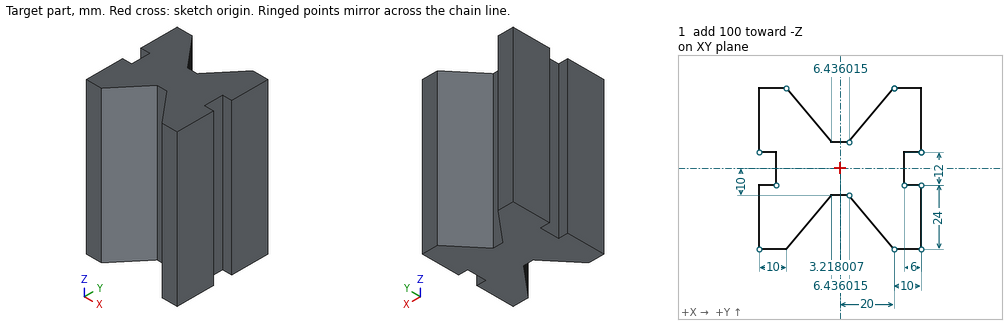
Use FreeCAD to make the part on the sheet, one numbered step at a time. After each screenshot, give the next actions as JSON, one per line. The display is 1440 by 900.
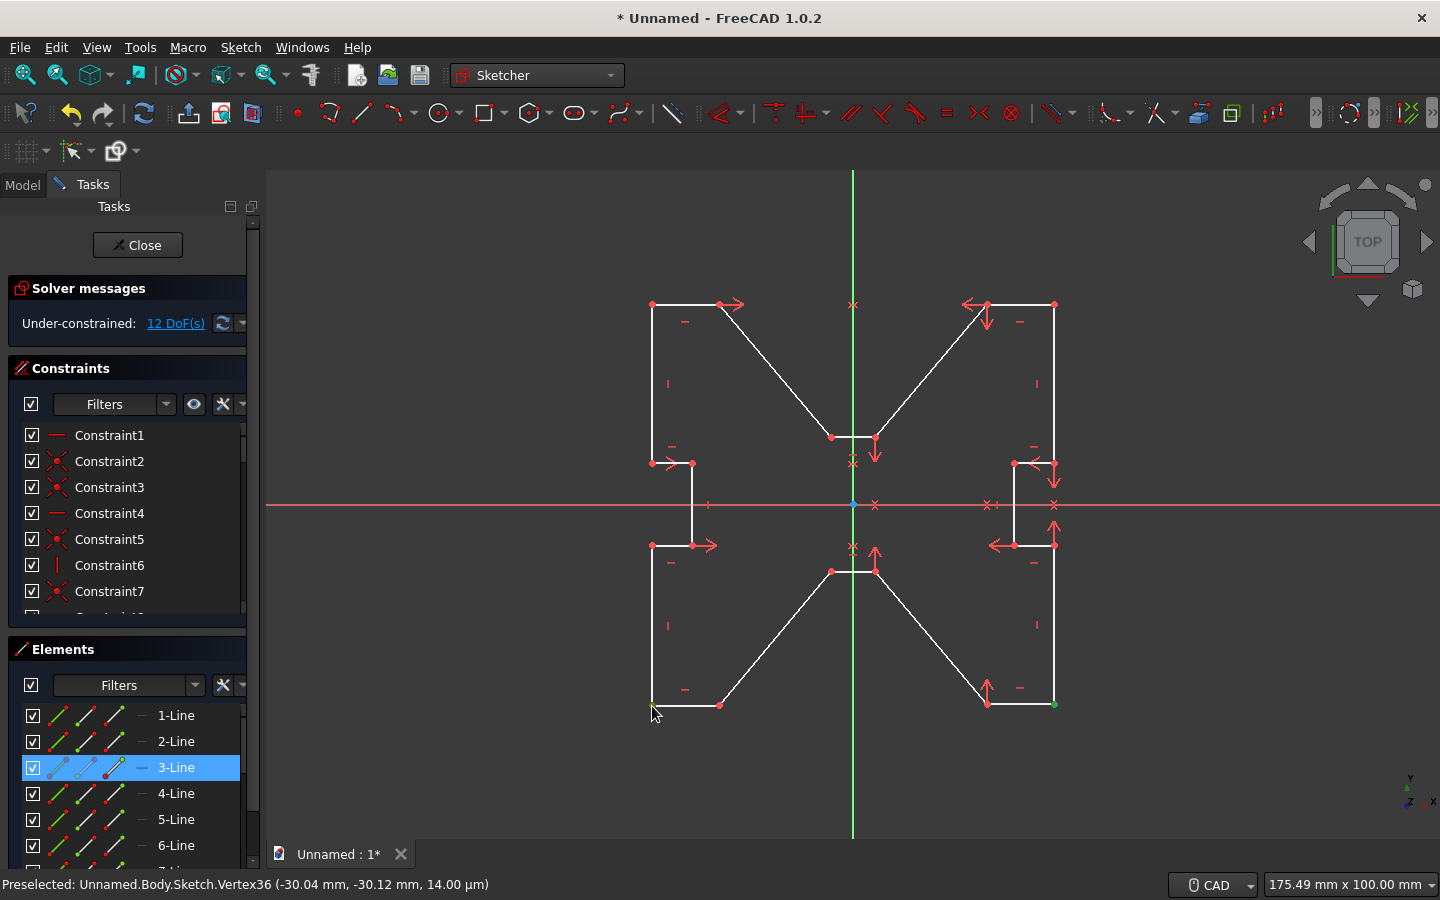
{"action": "left_click", "coordinate": [853, 767]}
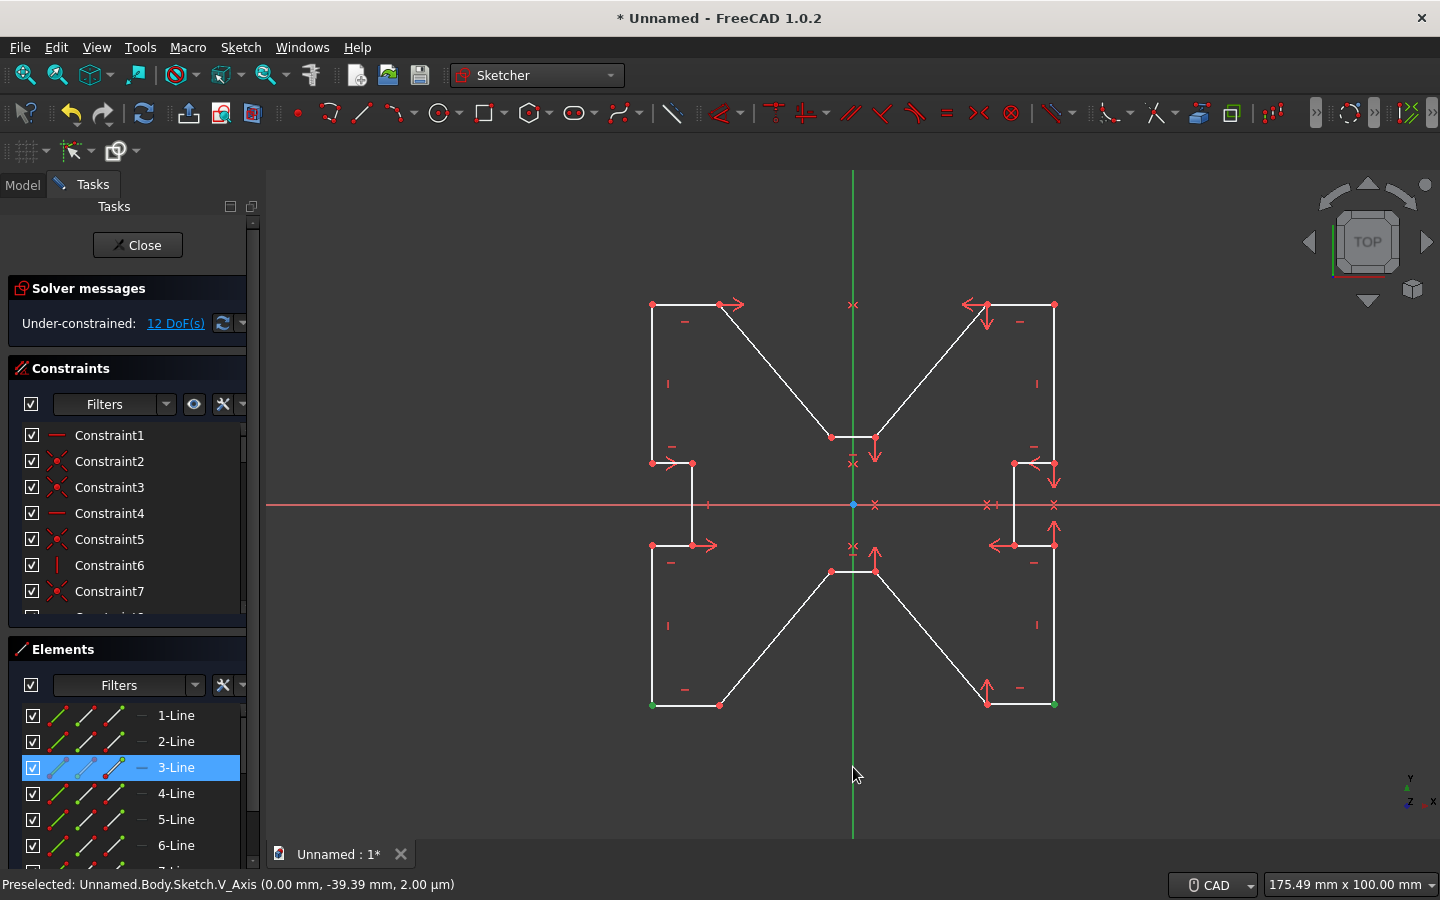
{"action": "key", "text": "s"}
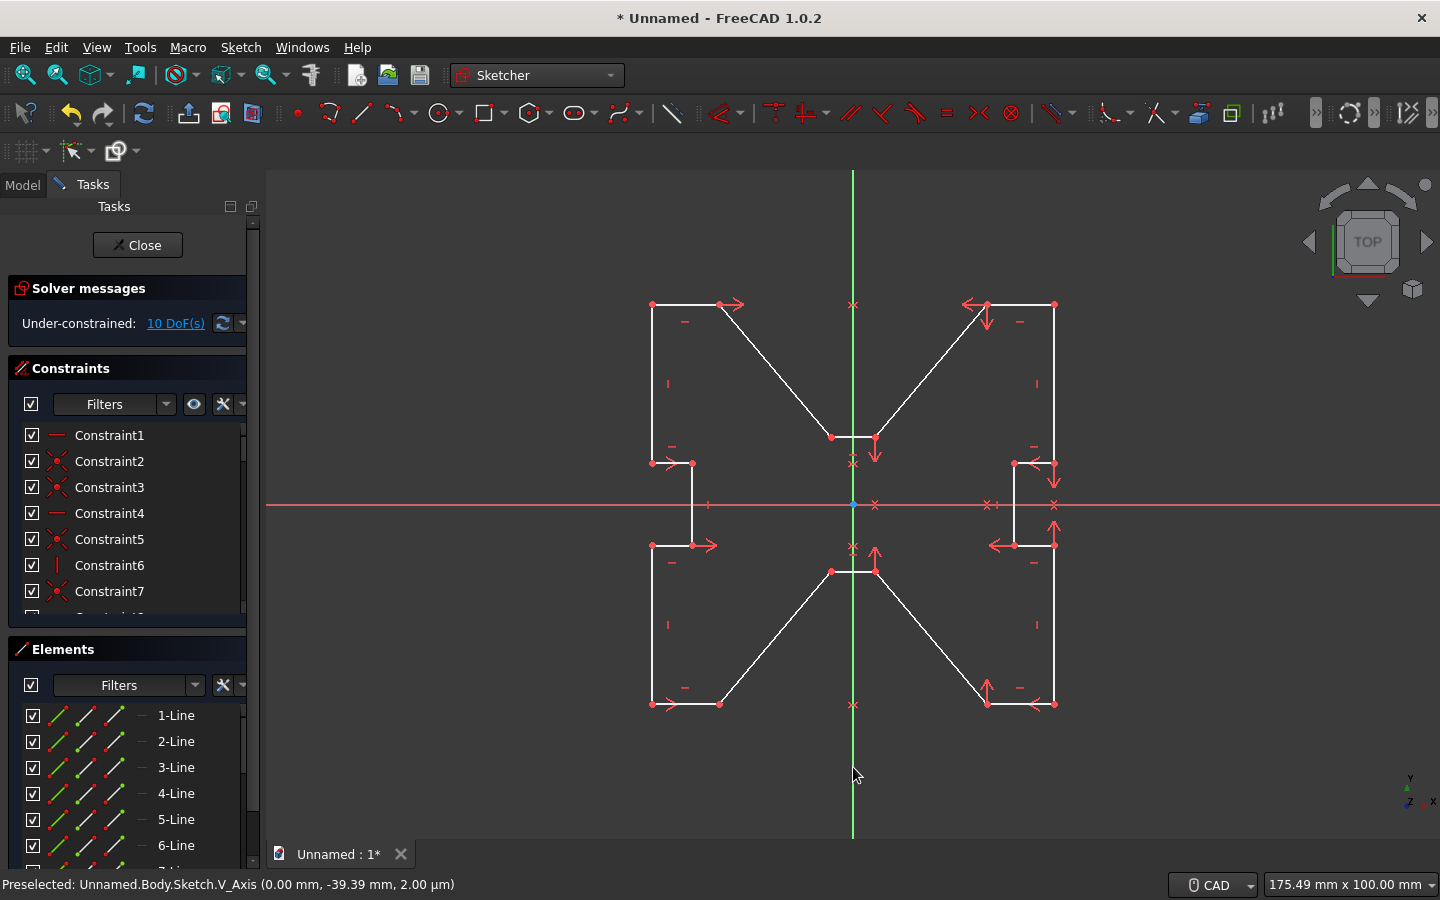
{"action": "left_click", "coordinate": [720, 114]}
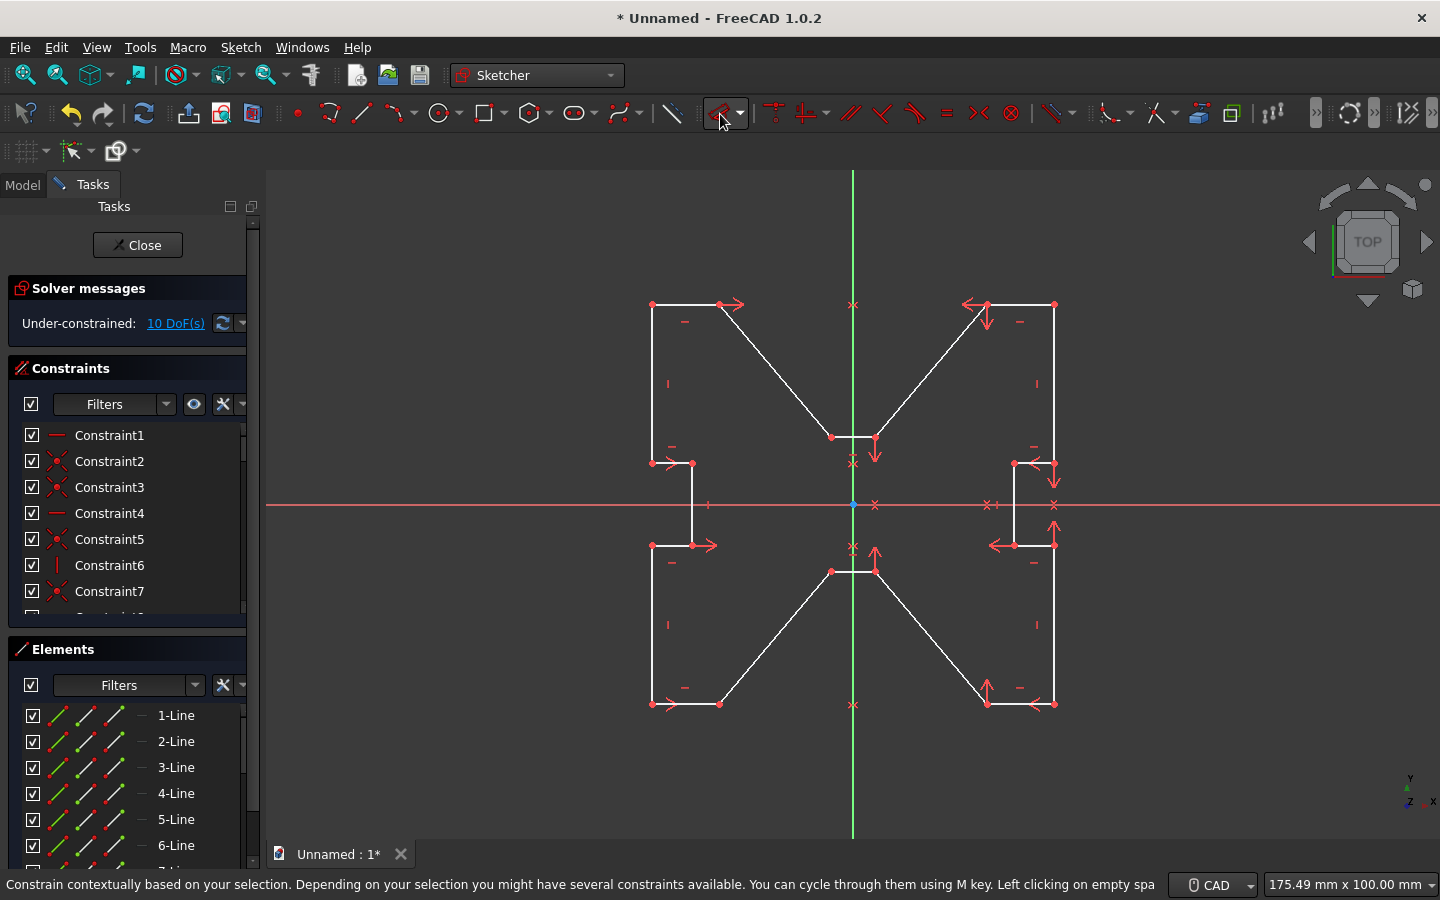
{"action": "left_click", "coordinate": [1042, 546]}
{"action": "left_click", "coordinate": [1034, 580]}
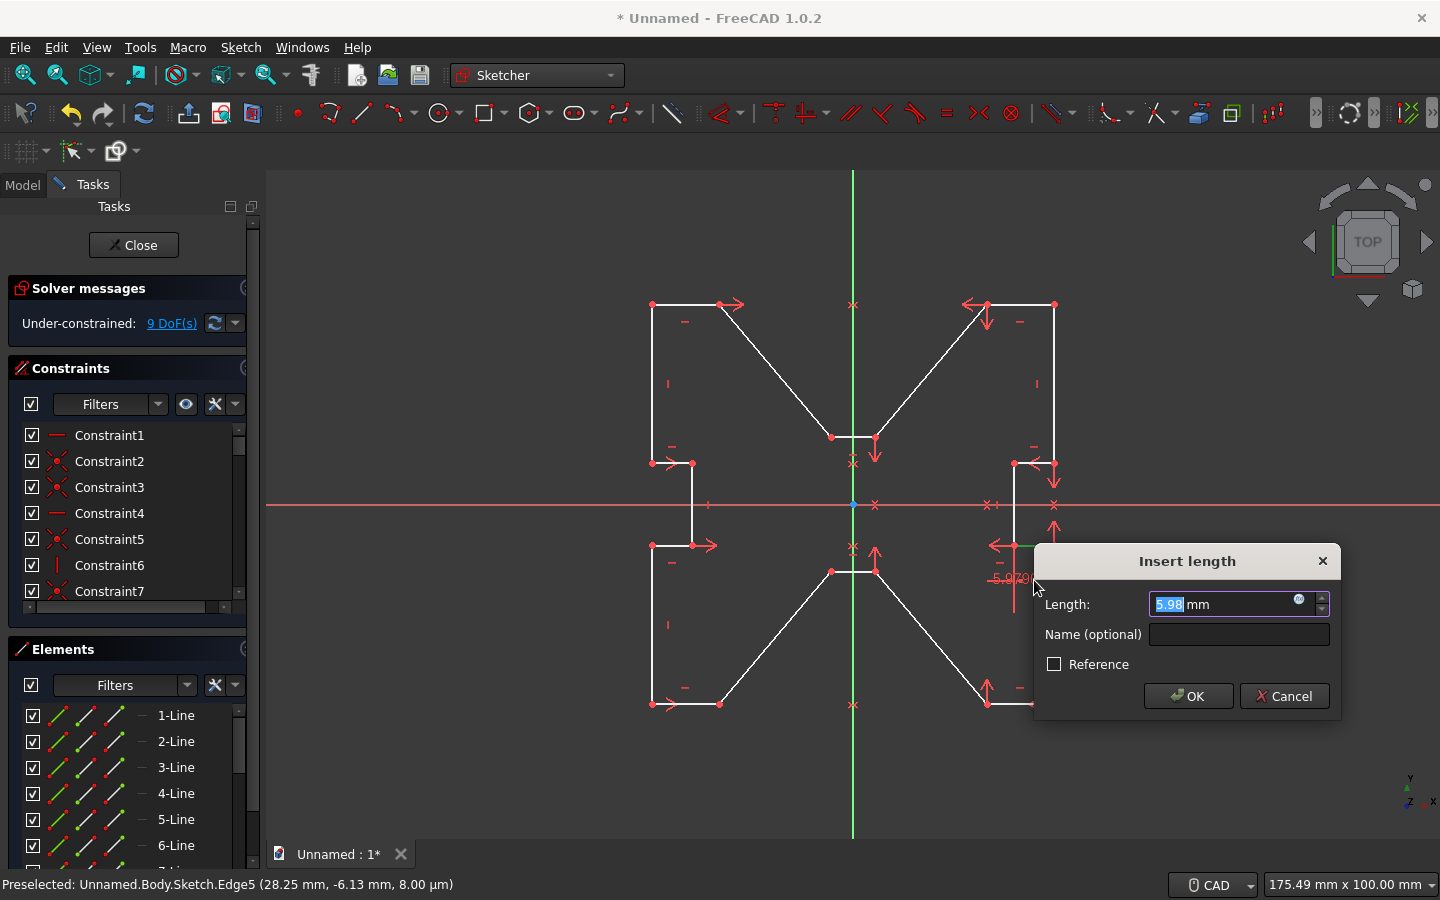
{"action": "type", "text": "6"}
{"action": "key", "text": "Return"}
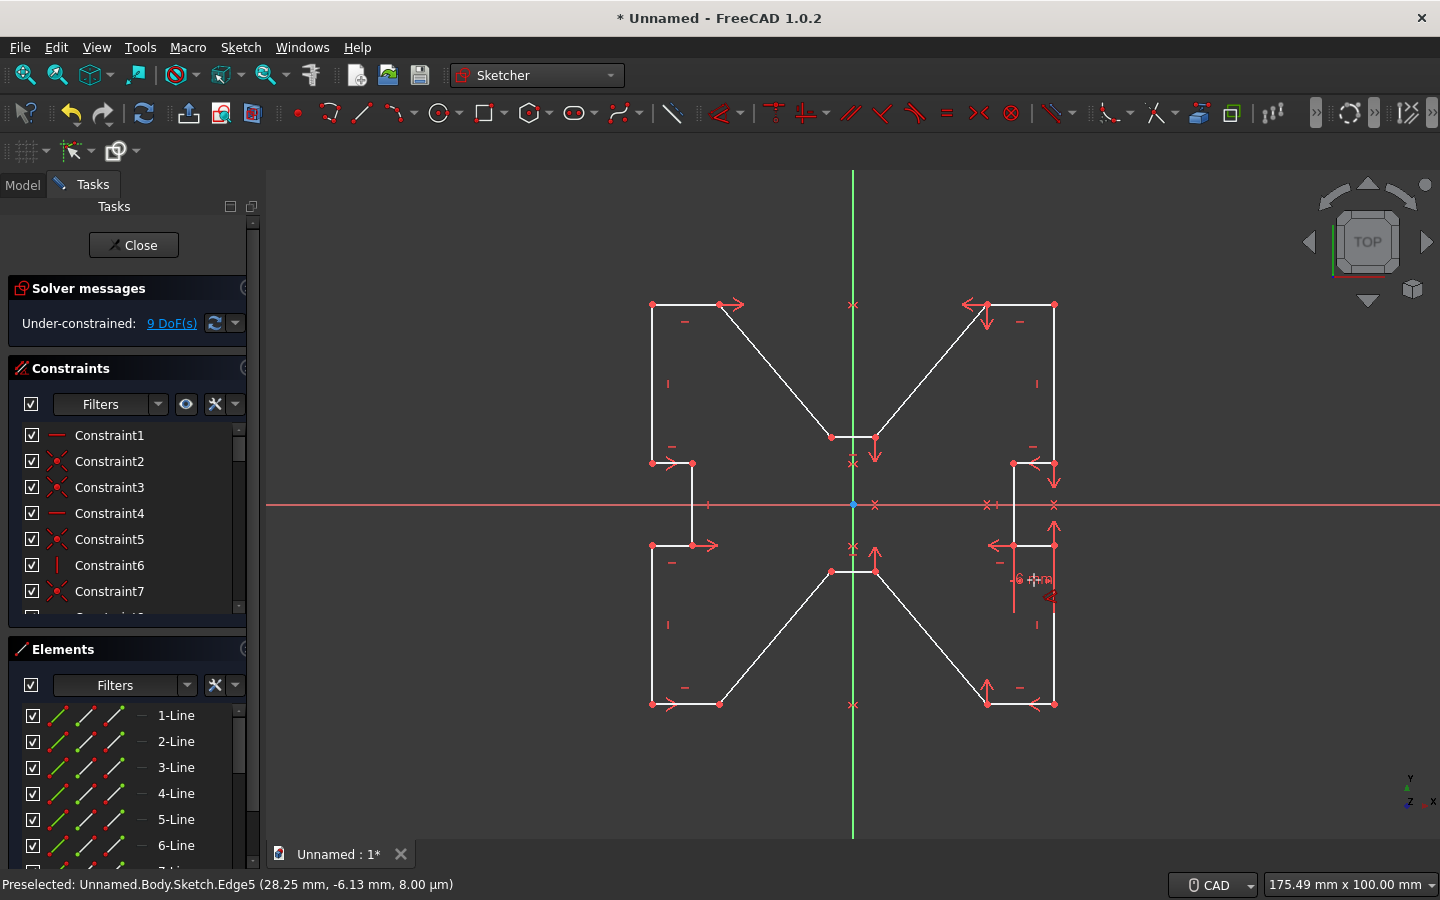
{"action": "left_click", "coordinate": [1007, 704]}
{"action": "left_click", "coordinate": [1020, 738]}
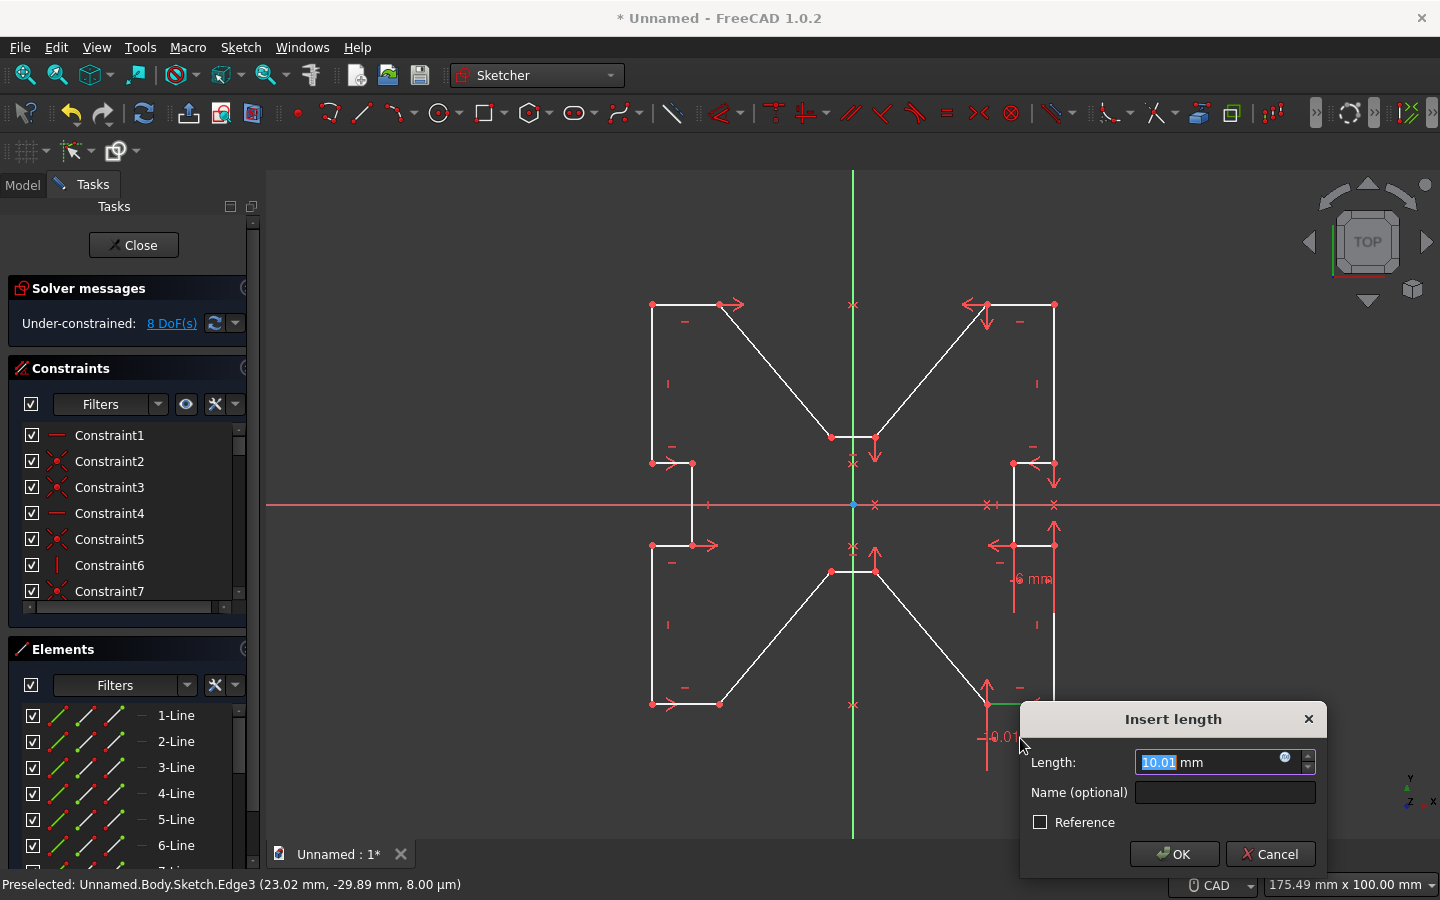
{"action": "type", "text": "10"}
{"action": "key", "text": "Return"}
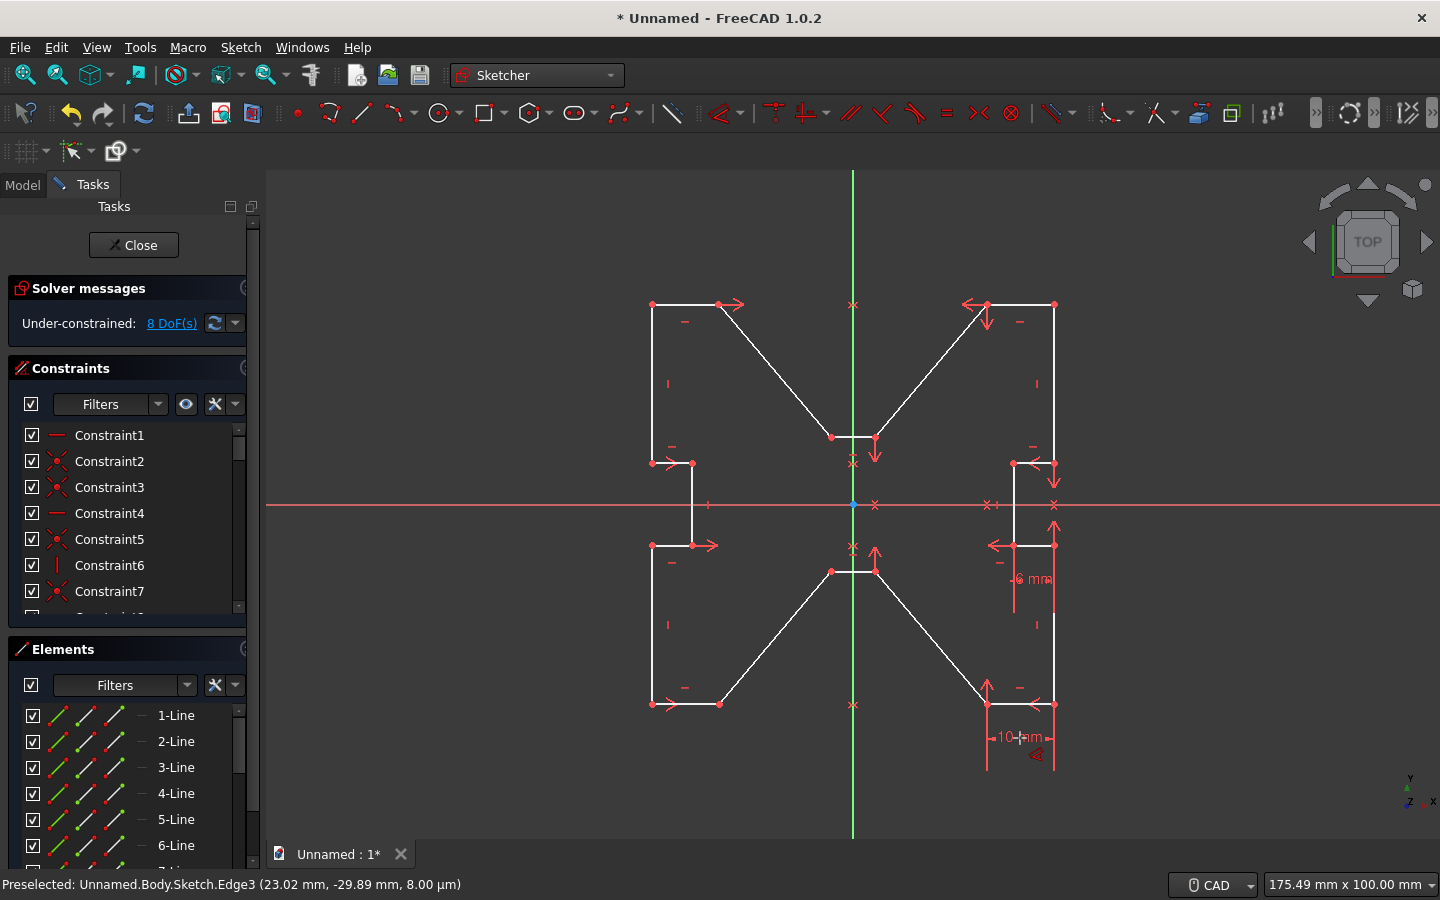
{"action": "left_click", "coordinate": [1054, 657]}
{"action": "left_click", "coordinate": [1088, 625]}